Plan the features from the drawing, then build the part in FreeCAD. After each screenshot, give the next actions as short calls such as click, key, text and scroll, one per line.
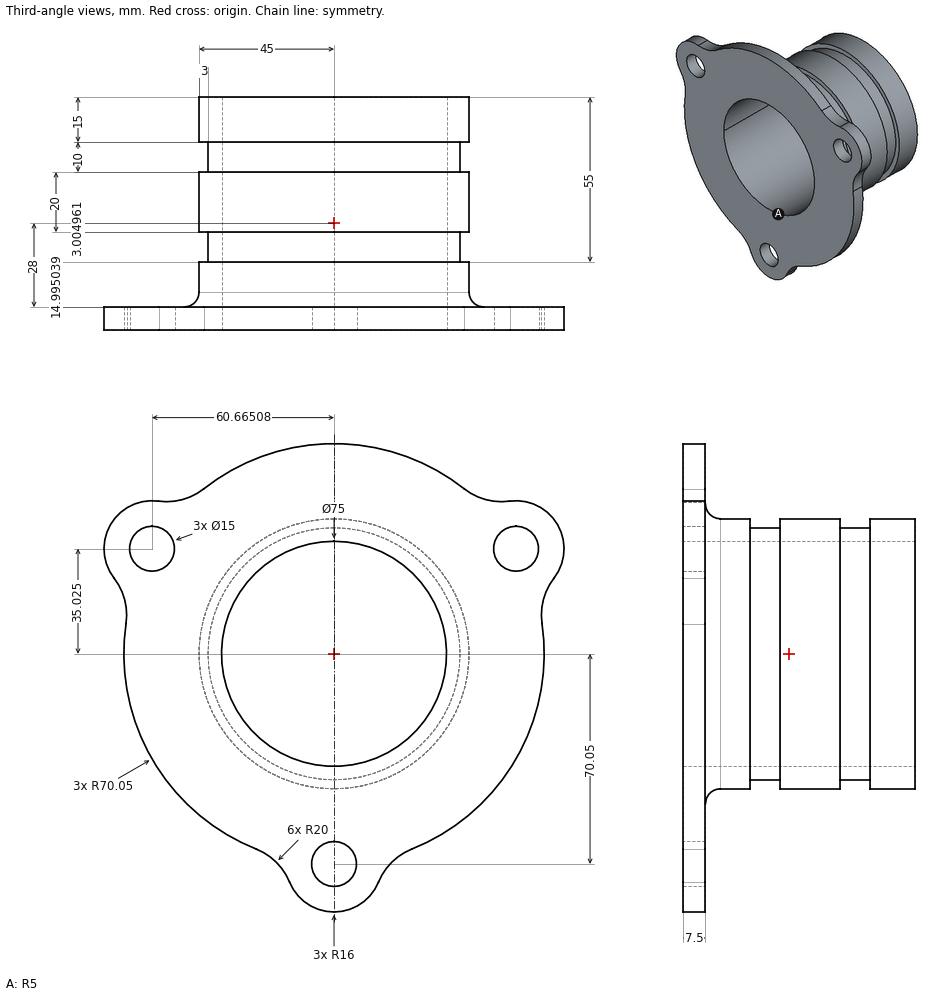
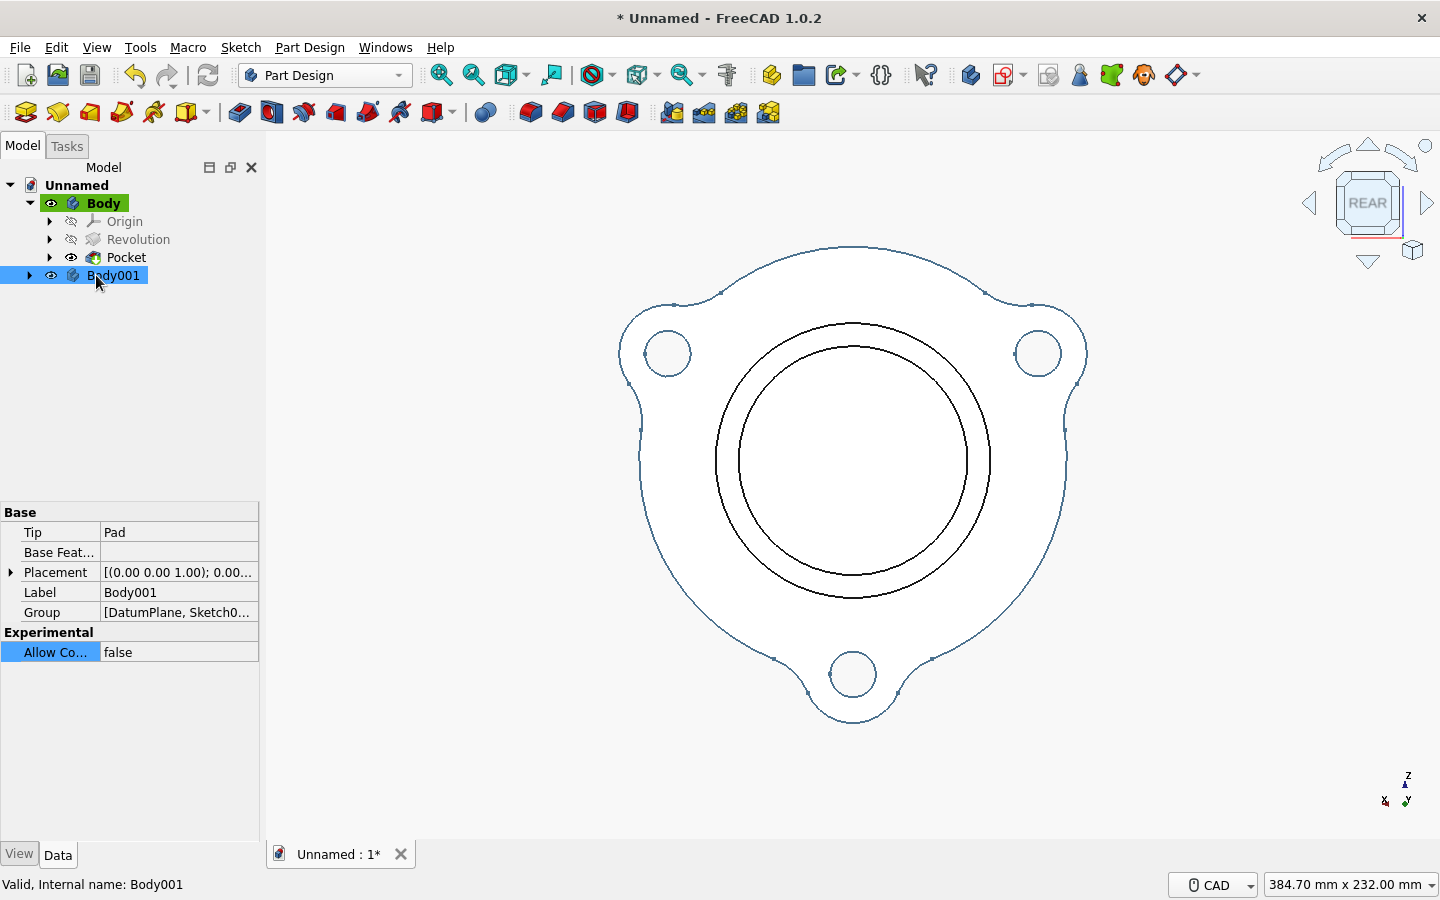
click(486, 112)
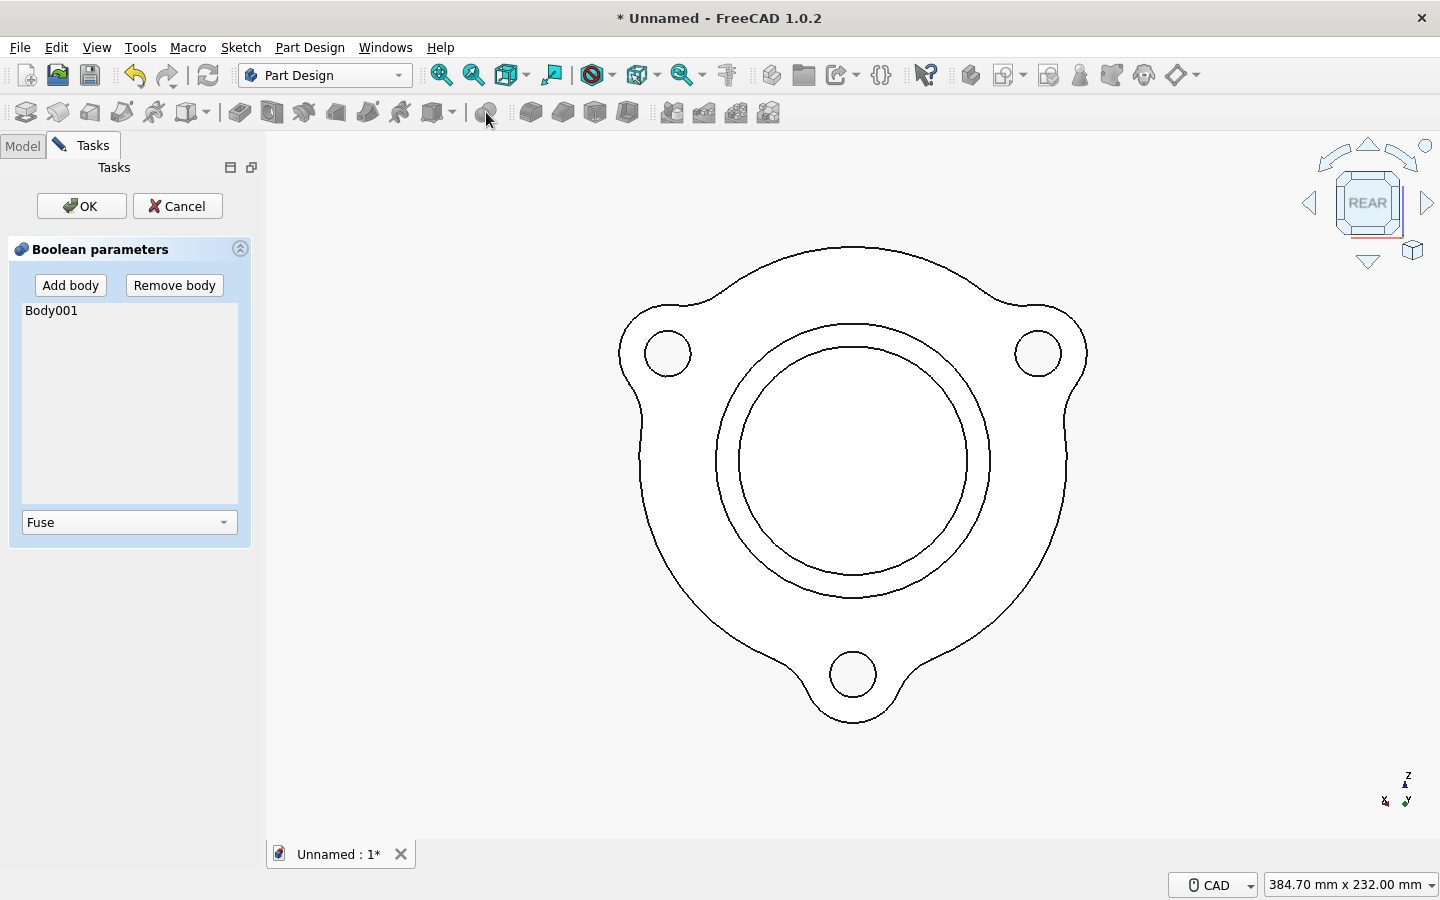
click(82, 206)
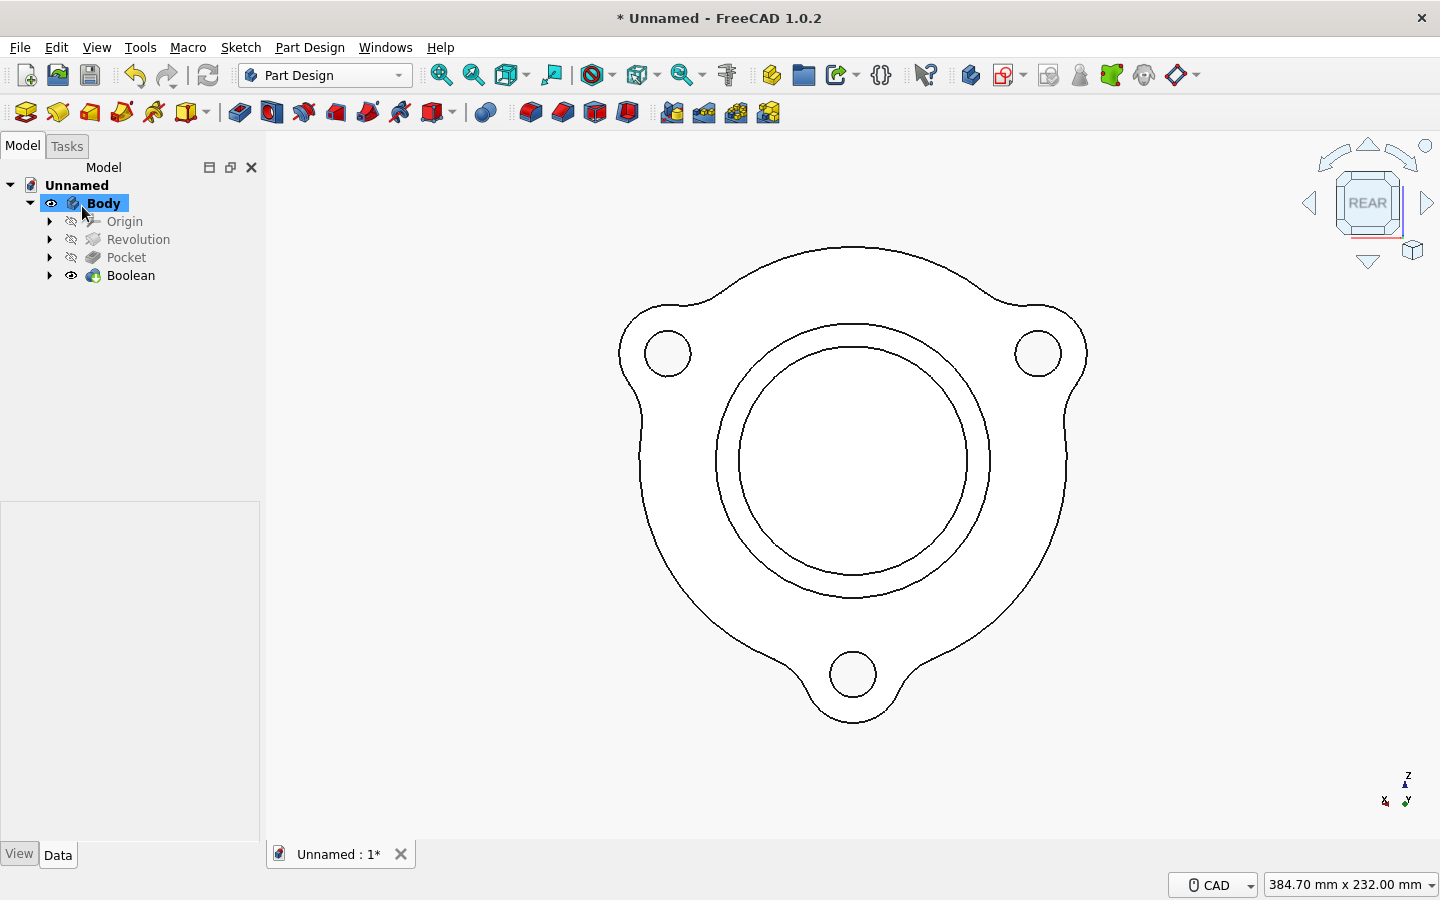
click(1004, 76)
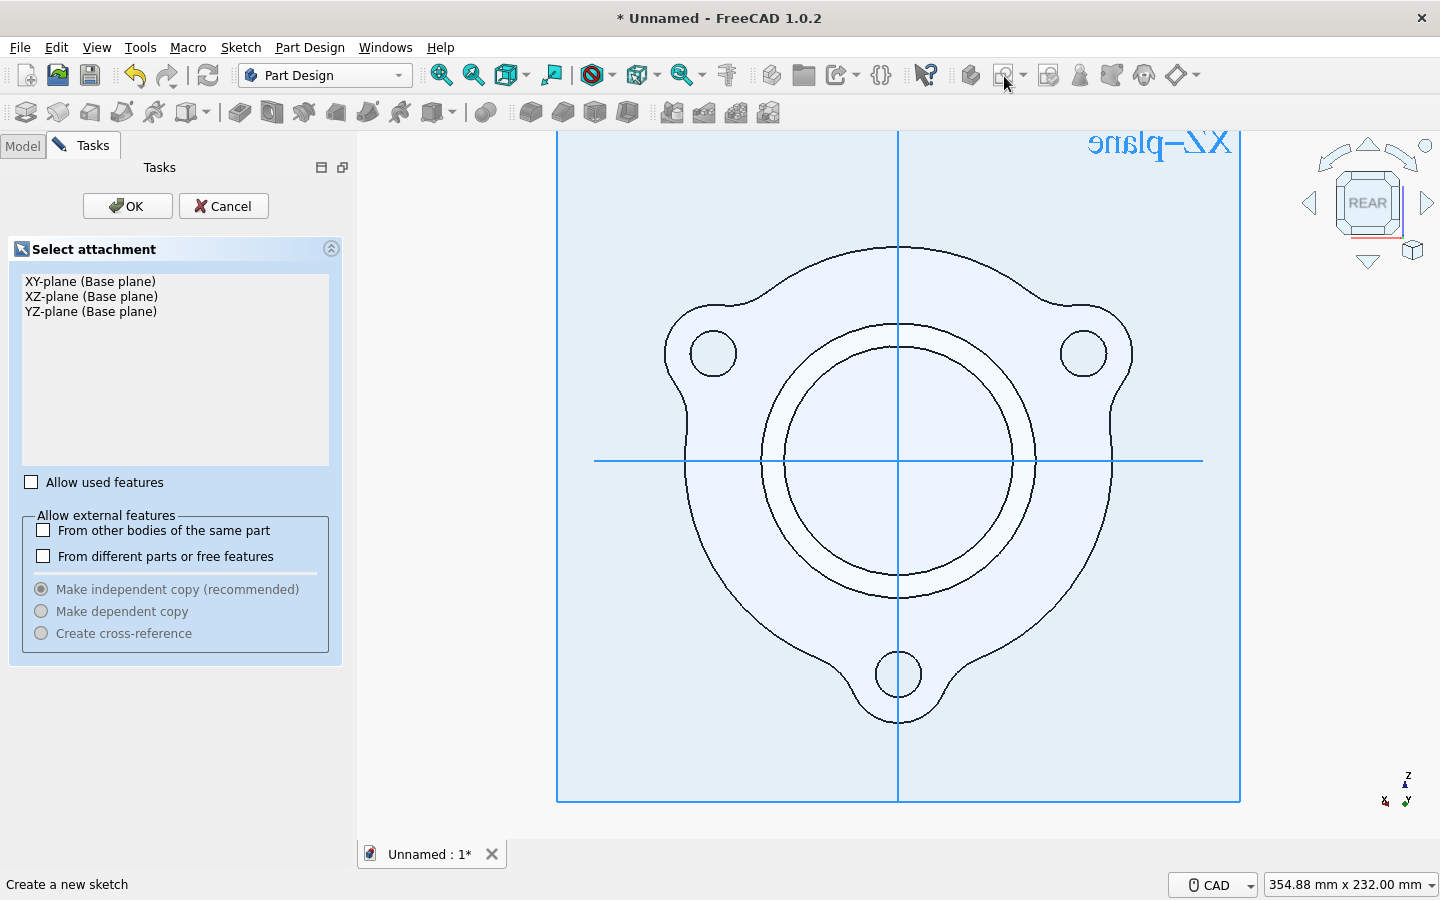
click(82, 282)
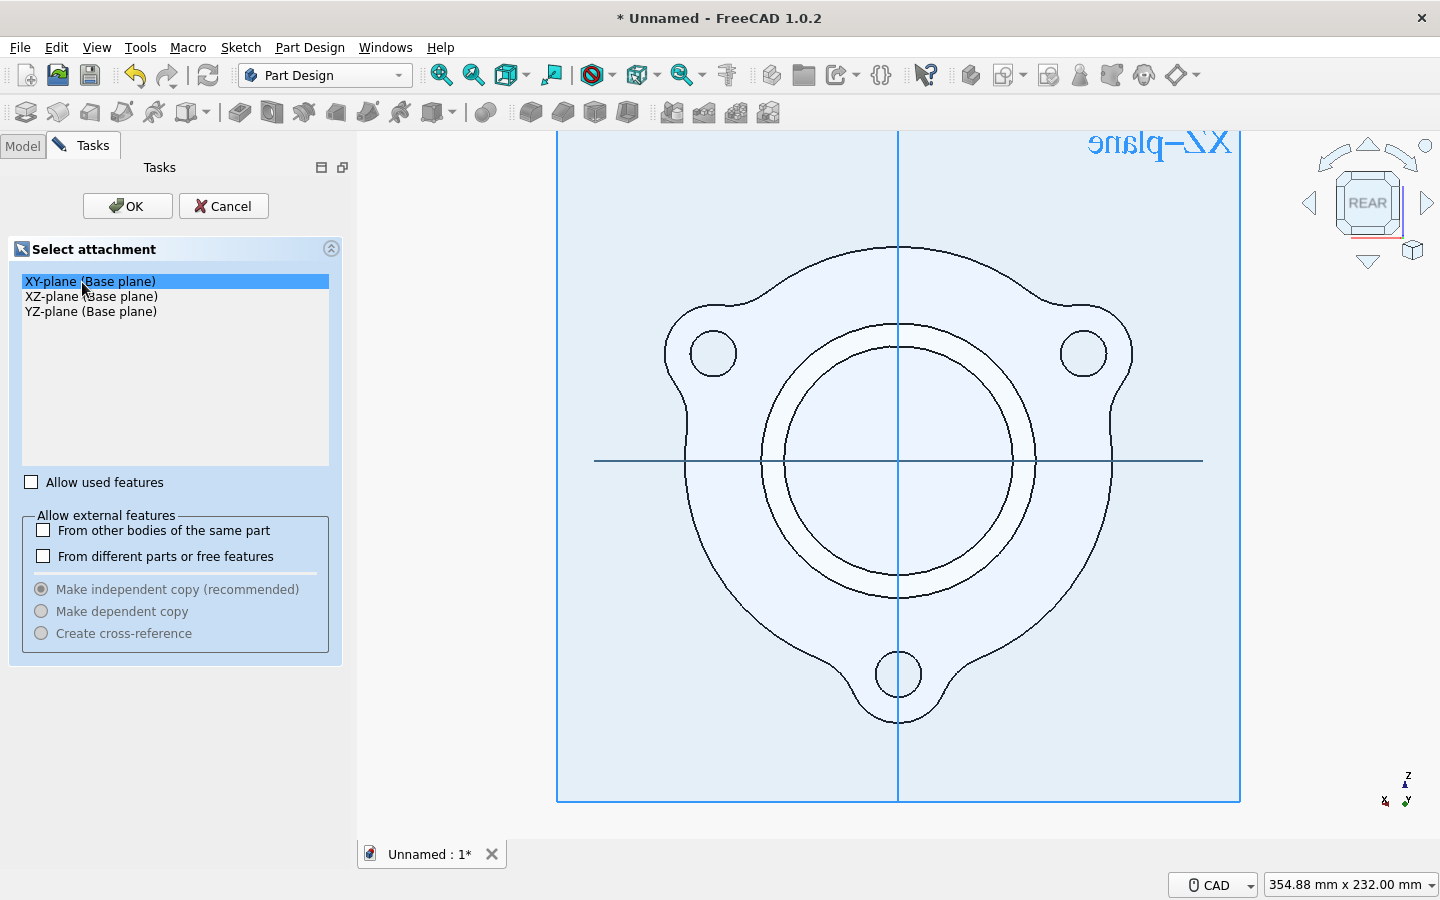
click(128, 206)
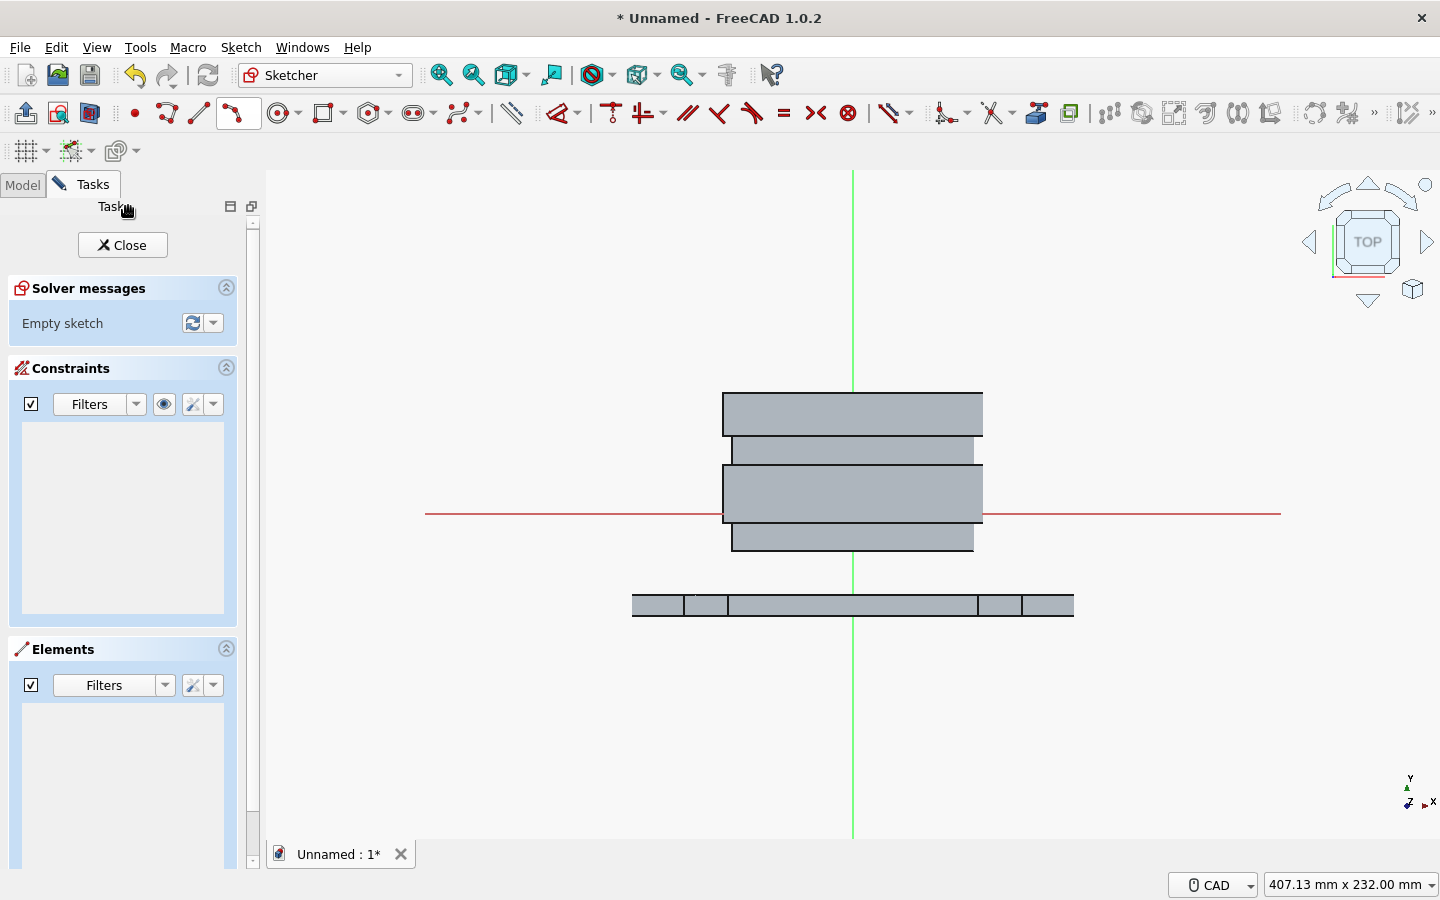
key(q)
key(s)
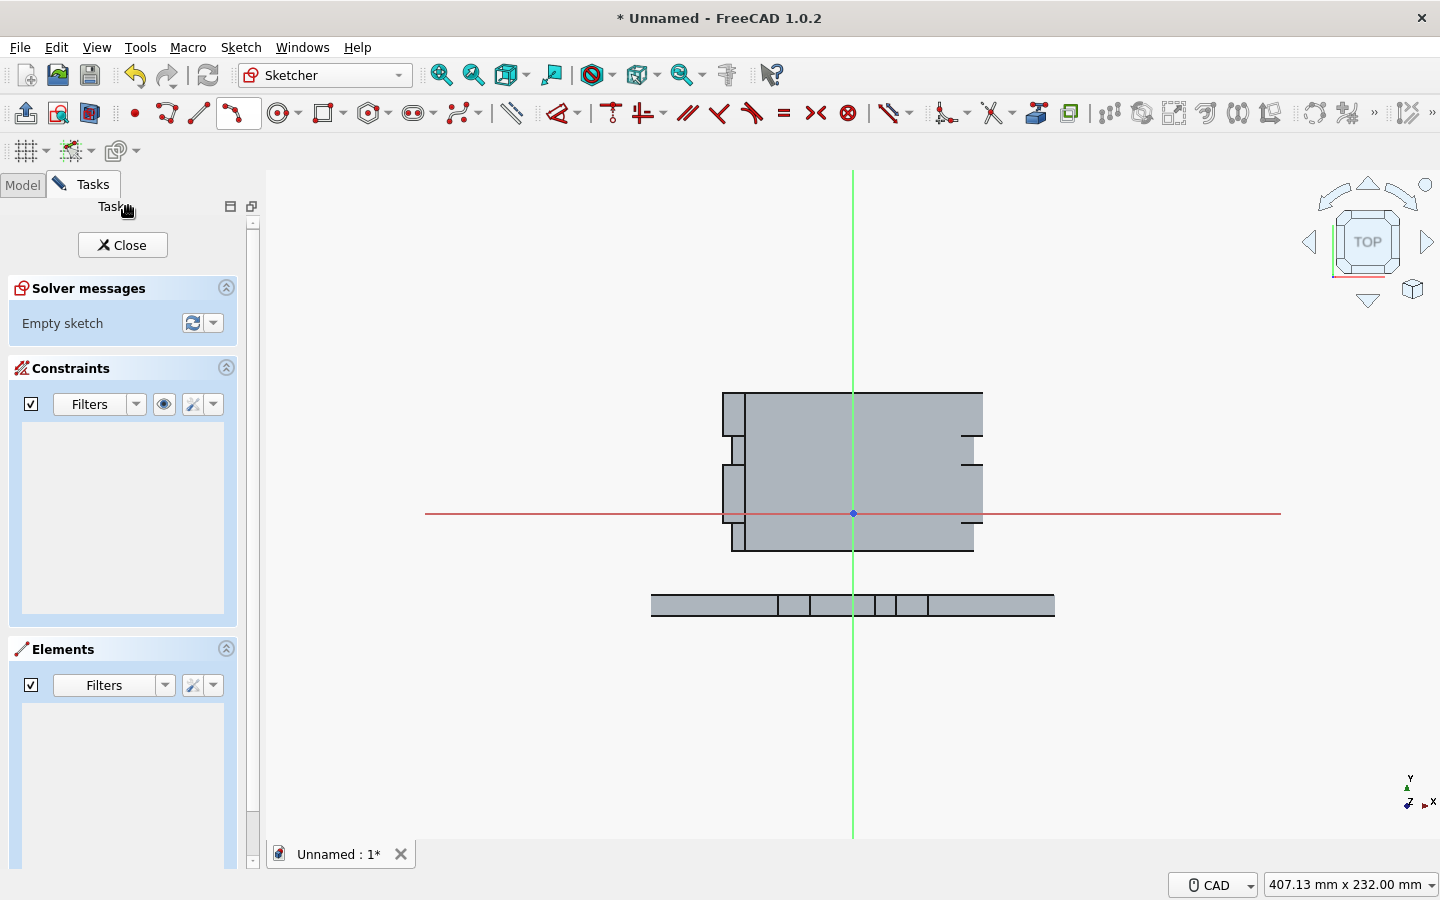
scroll(789, 567, up, 8)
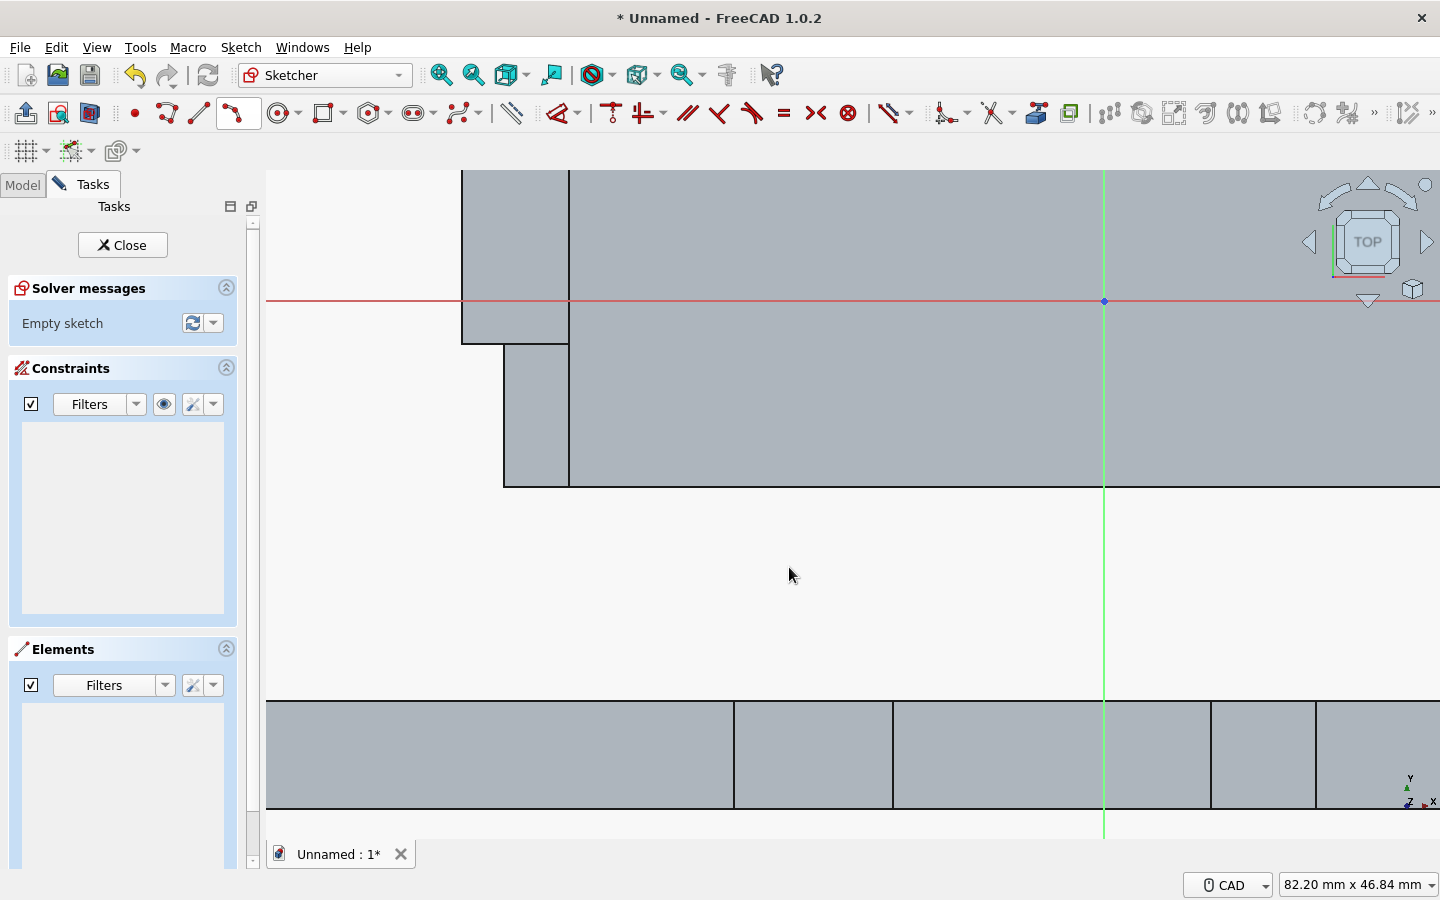
key(g)
key(r)